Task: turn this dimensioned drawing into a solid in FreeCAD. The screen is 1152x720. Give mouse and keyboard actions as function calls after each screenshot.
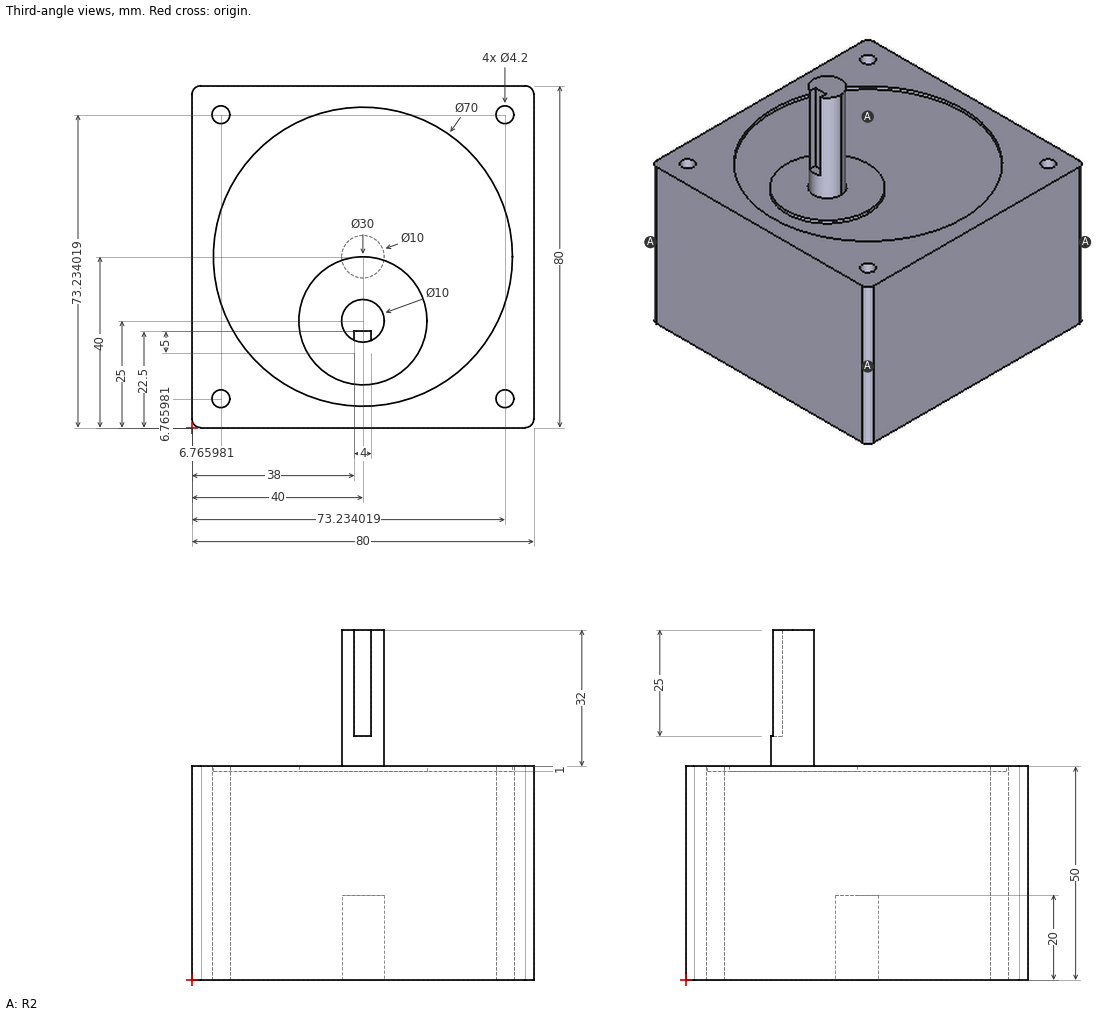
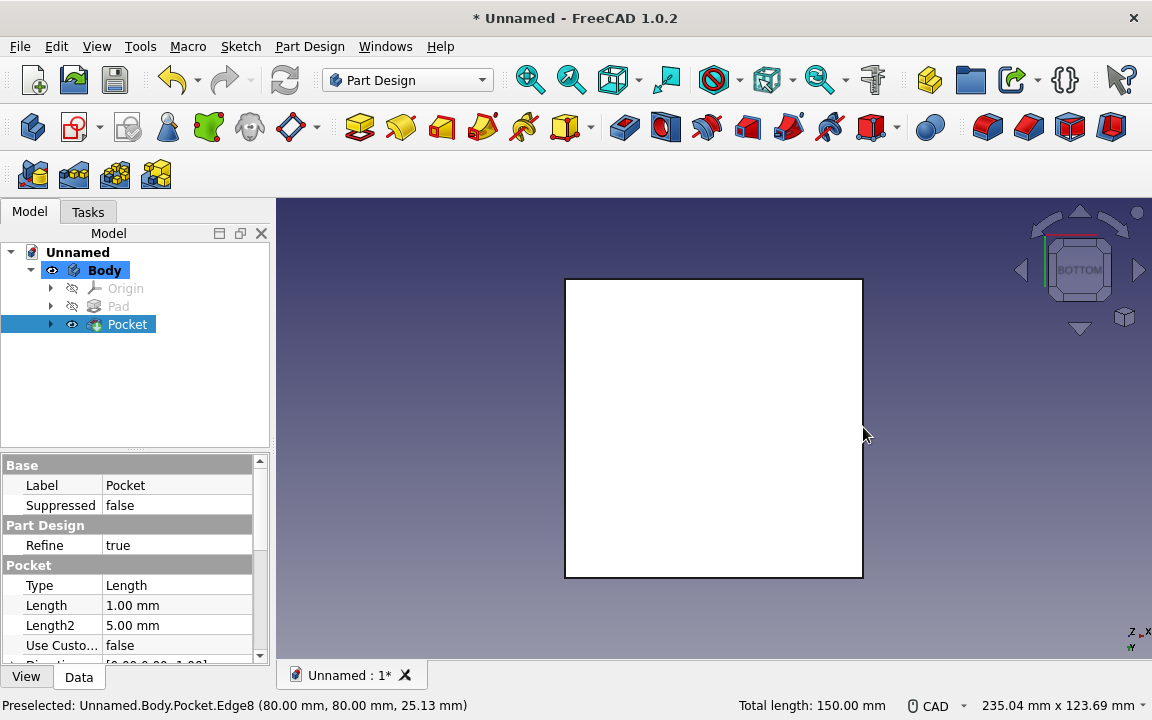
key(4)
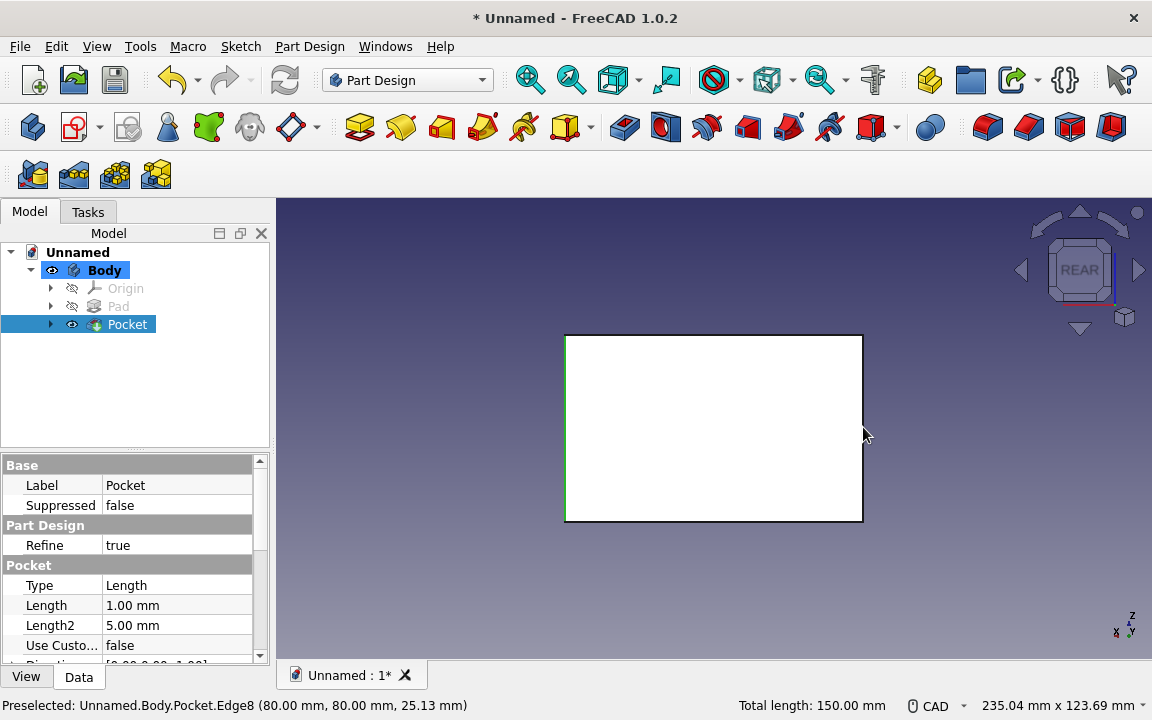
click(531, 80)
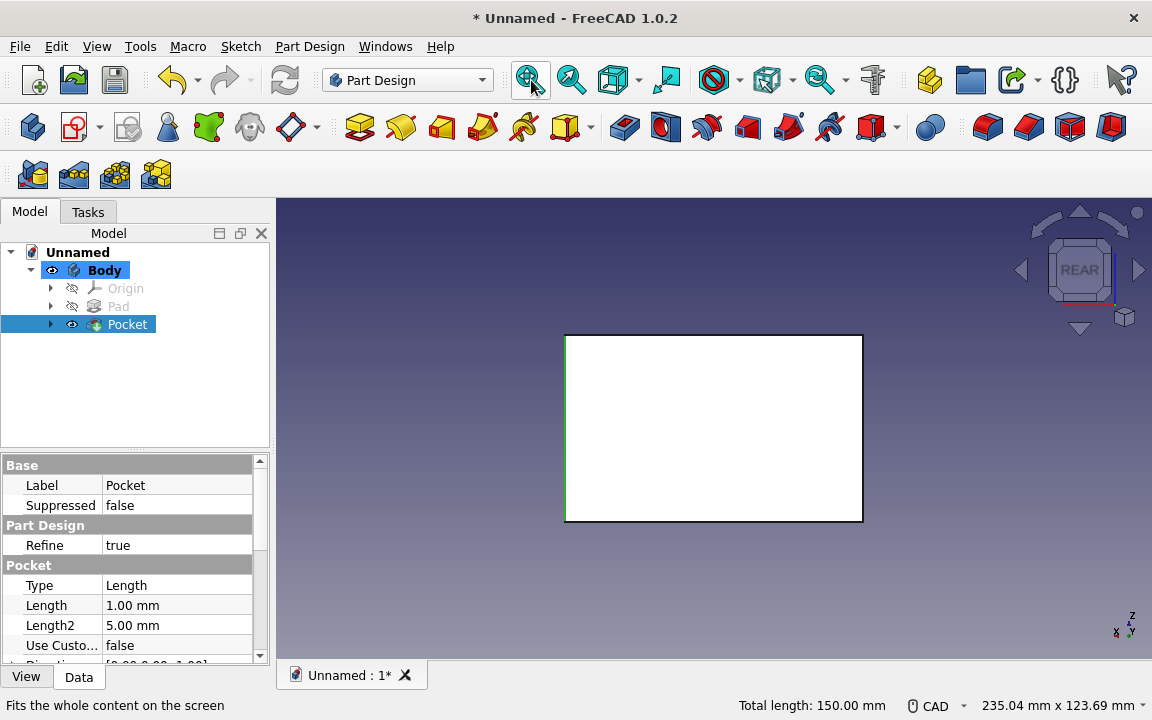
click(863, 428, ctrl)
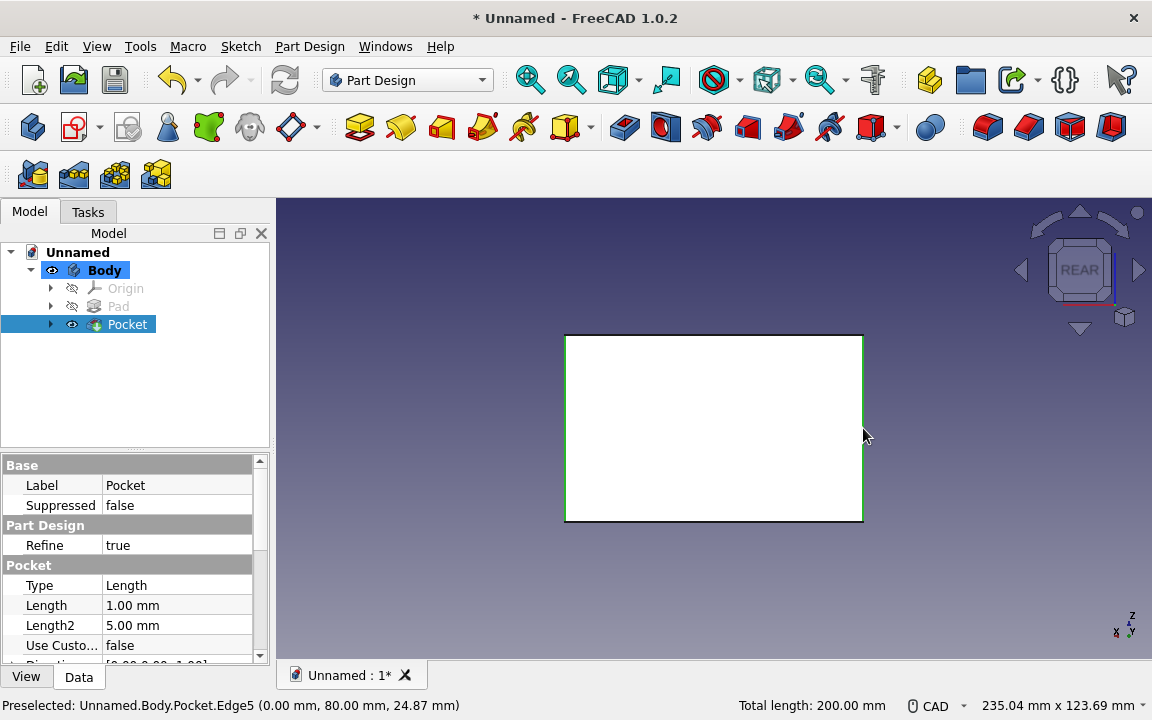
click(988, 128)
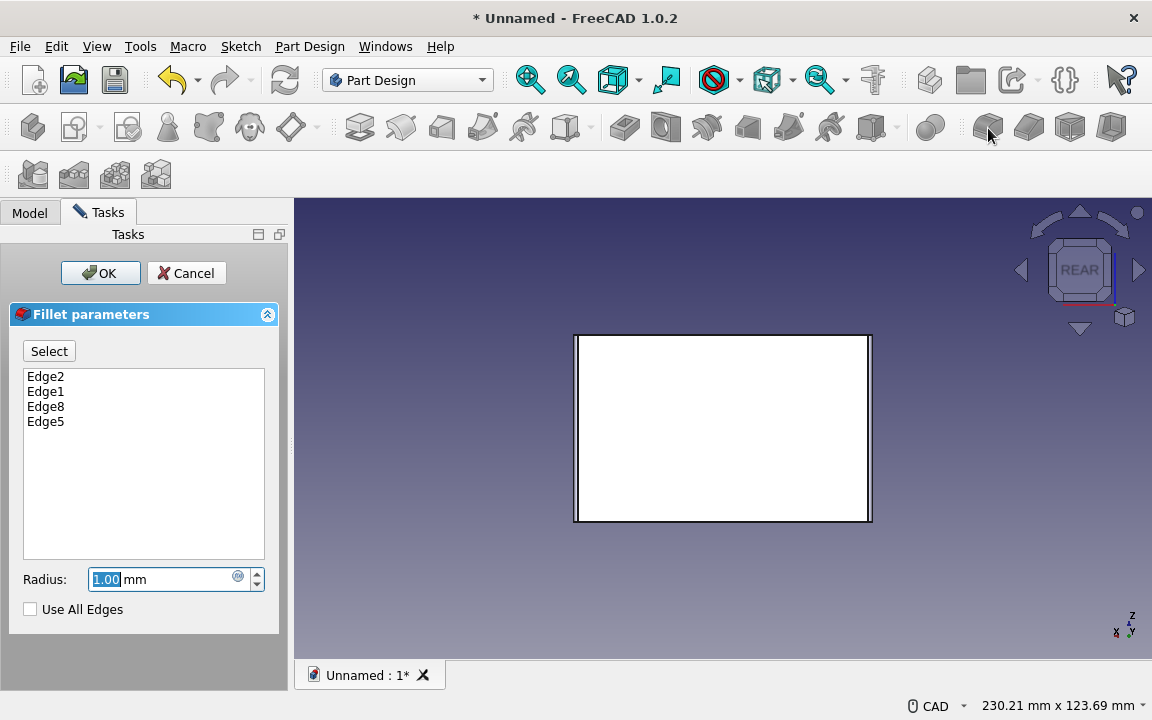
text(2)
key(Tab)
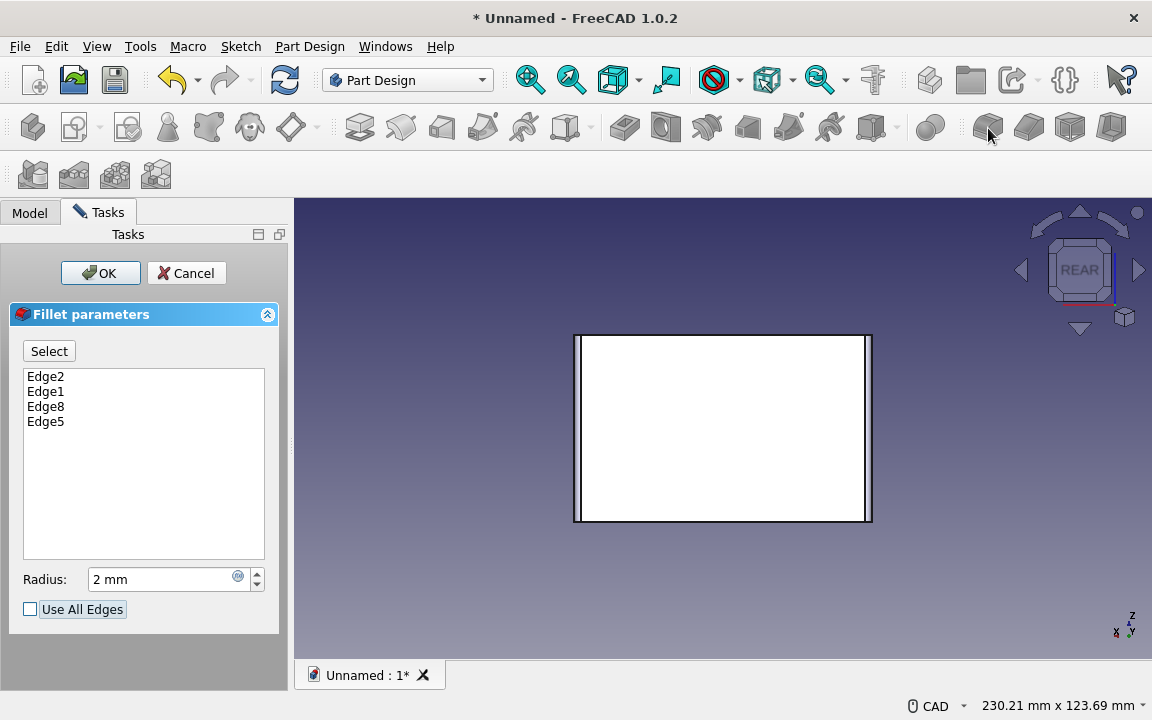
click(101, 273)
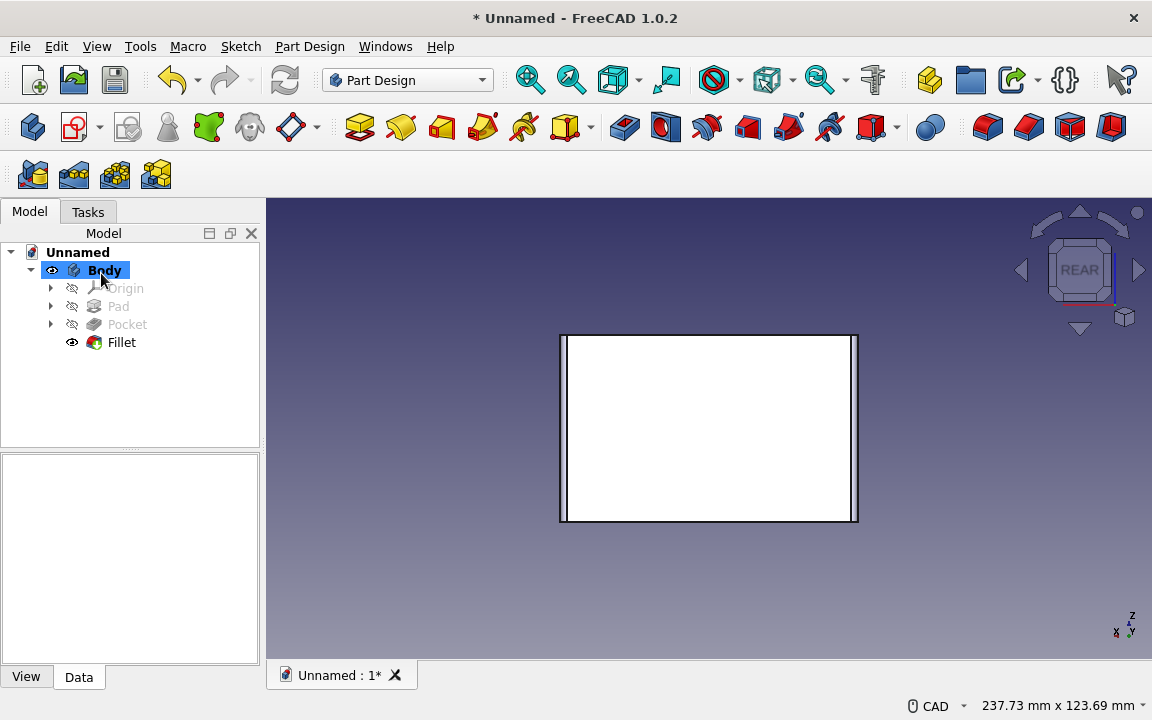
click(531, 80)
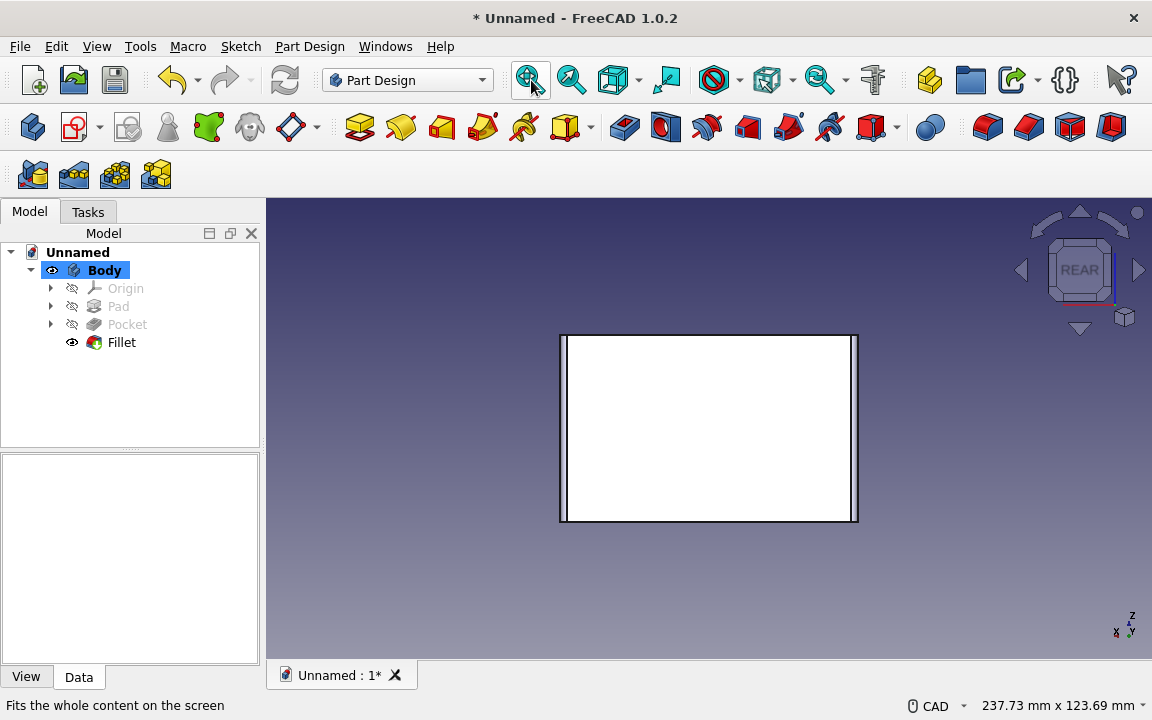
click(74, 128)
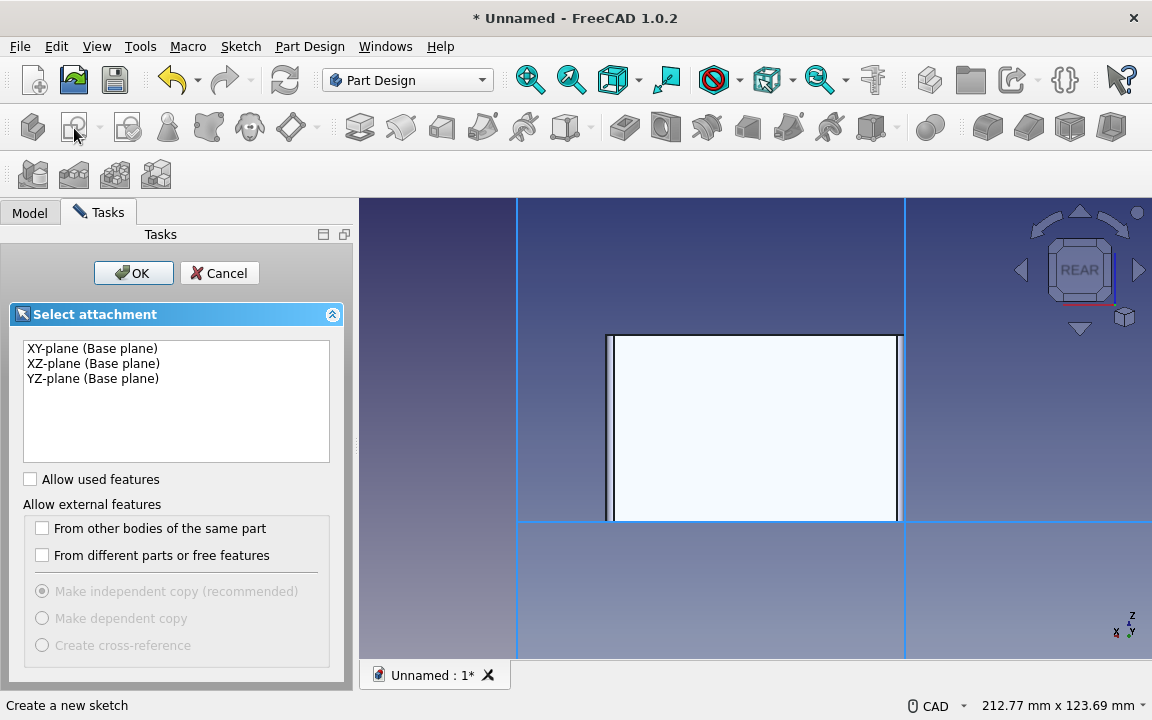
click(84, 348)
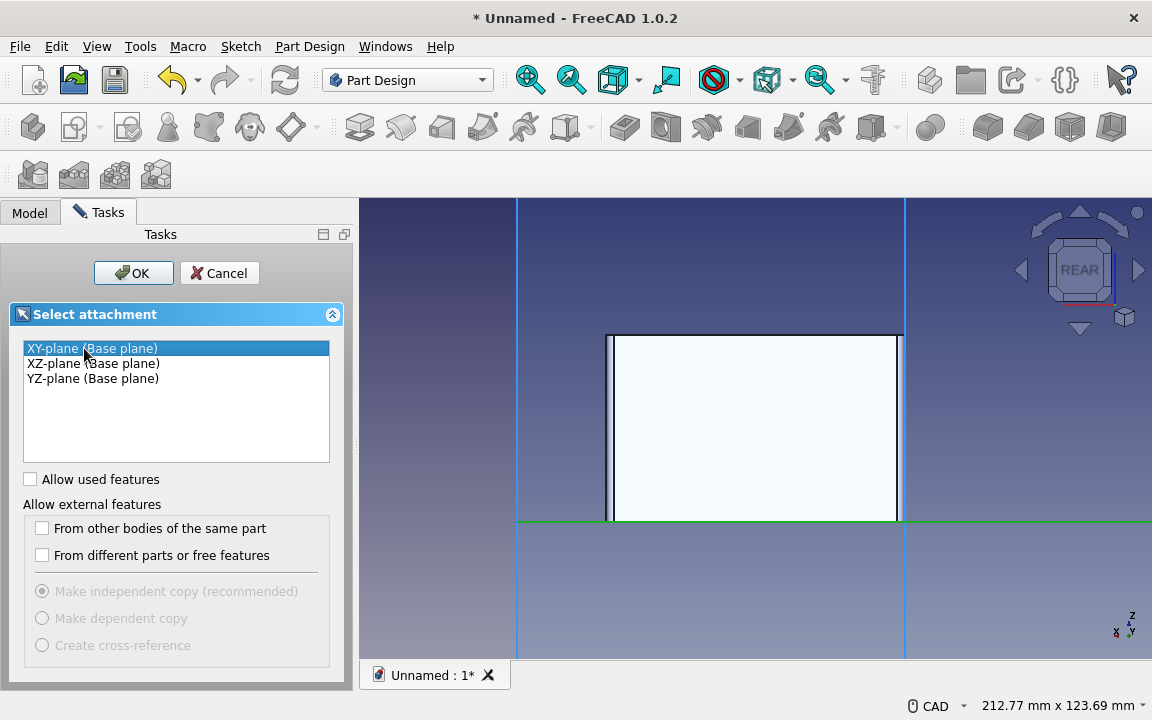
click(134, 273)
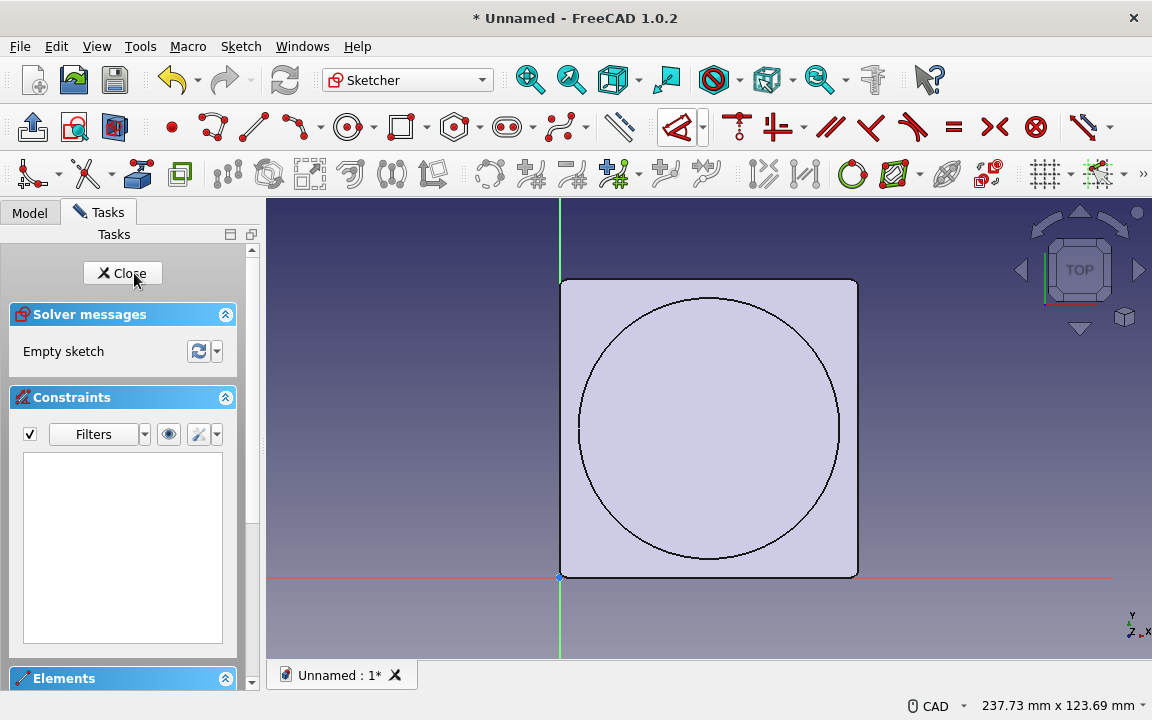
key(q)
key(s)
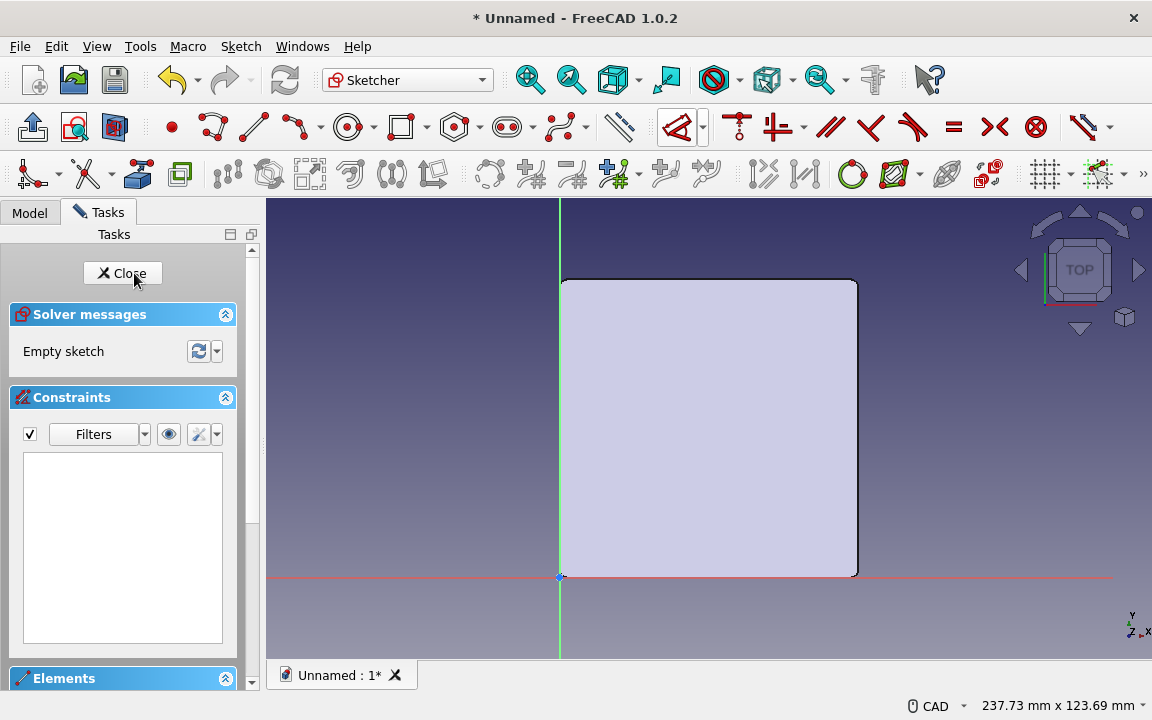
key(g)
key(c)